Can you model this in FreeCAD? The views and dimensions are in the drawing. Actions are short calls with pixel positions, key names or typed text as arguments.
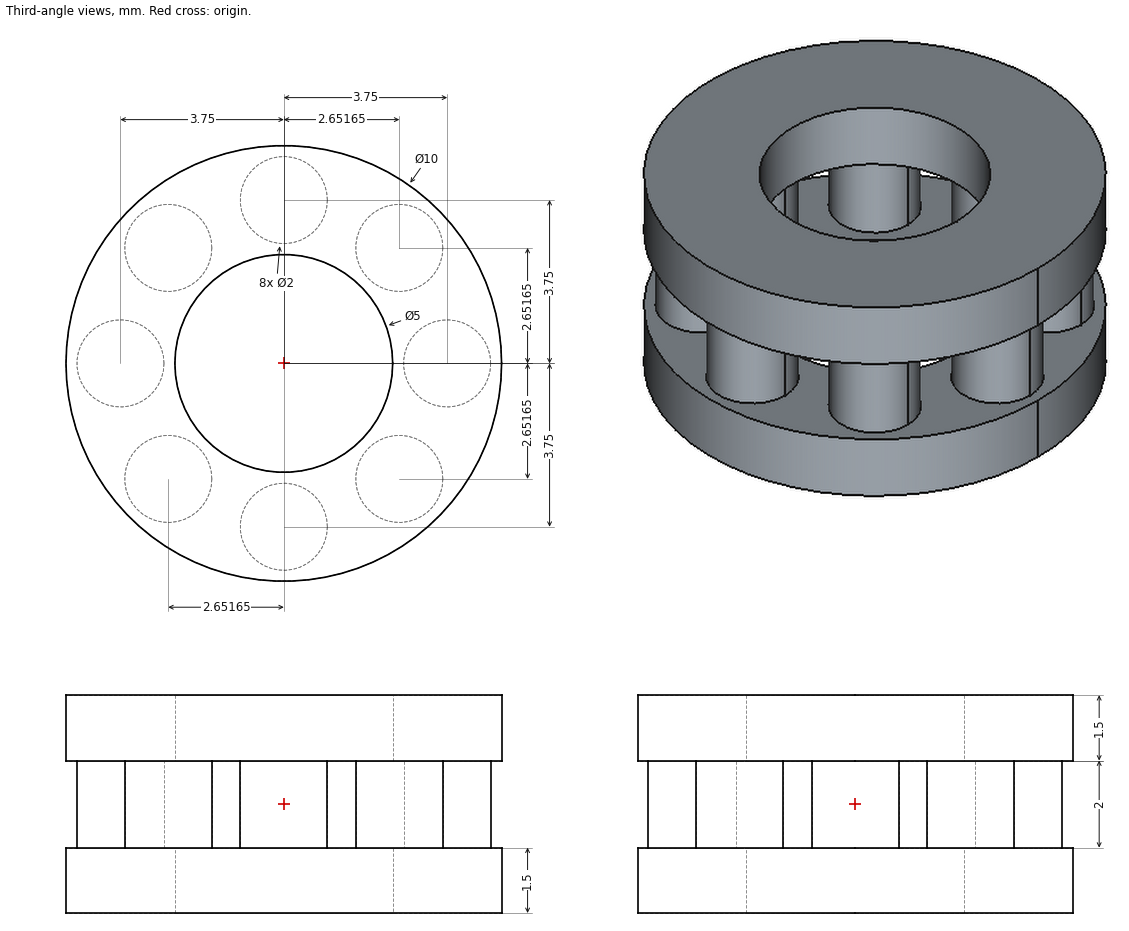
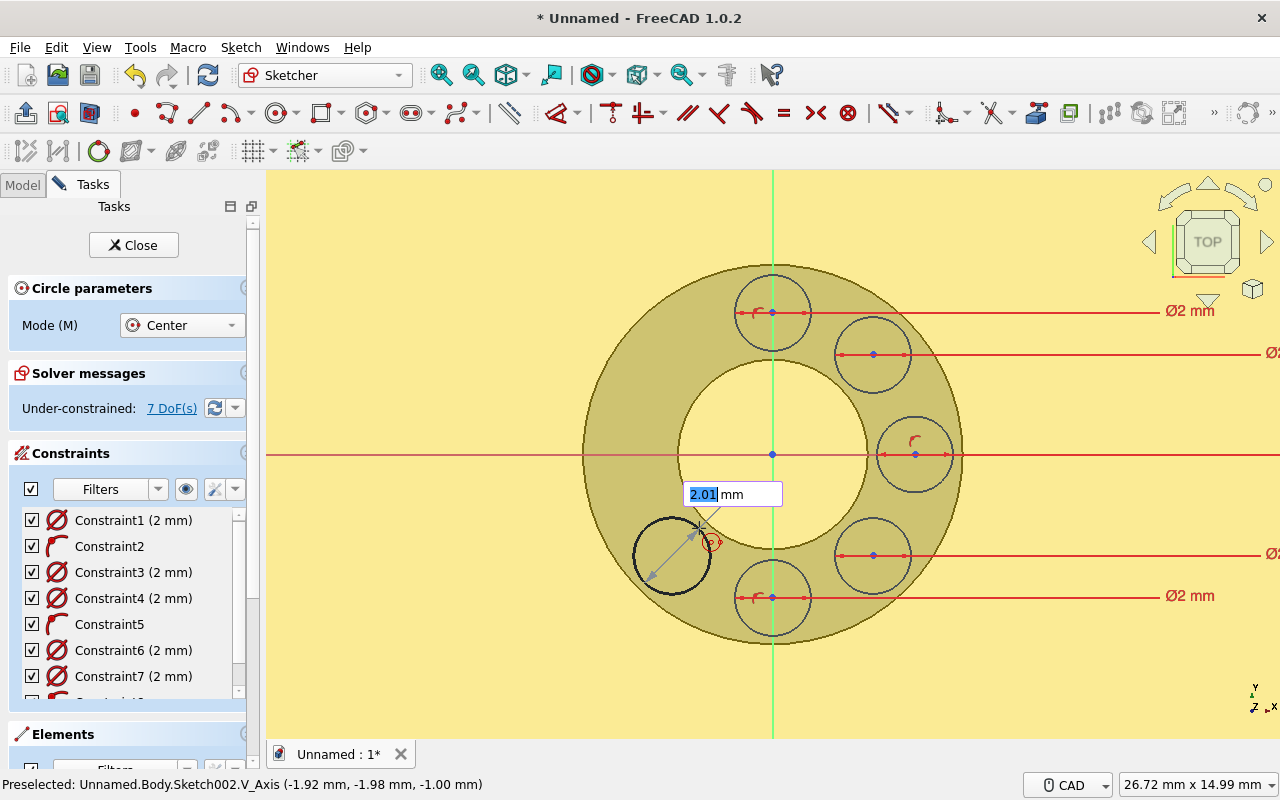
text(2)
key(Return)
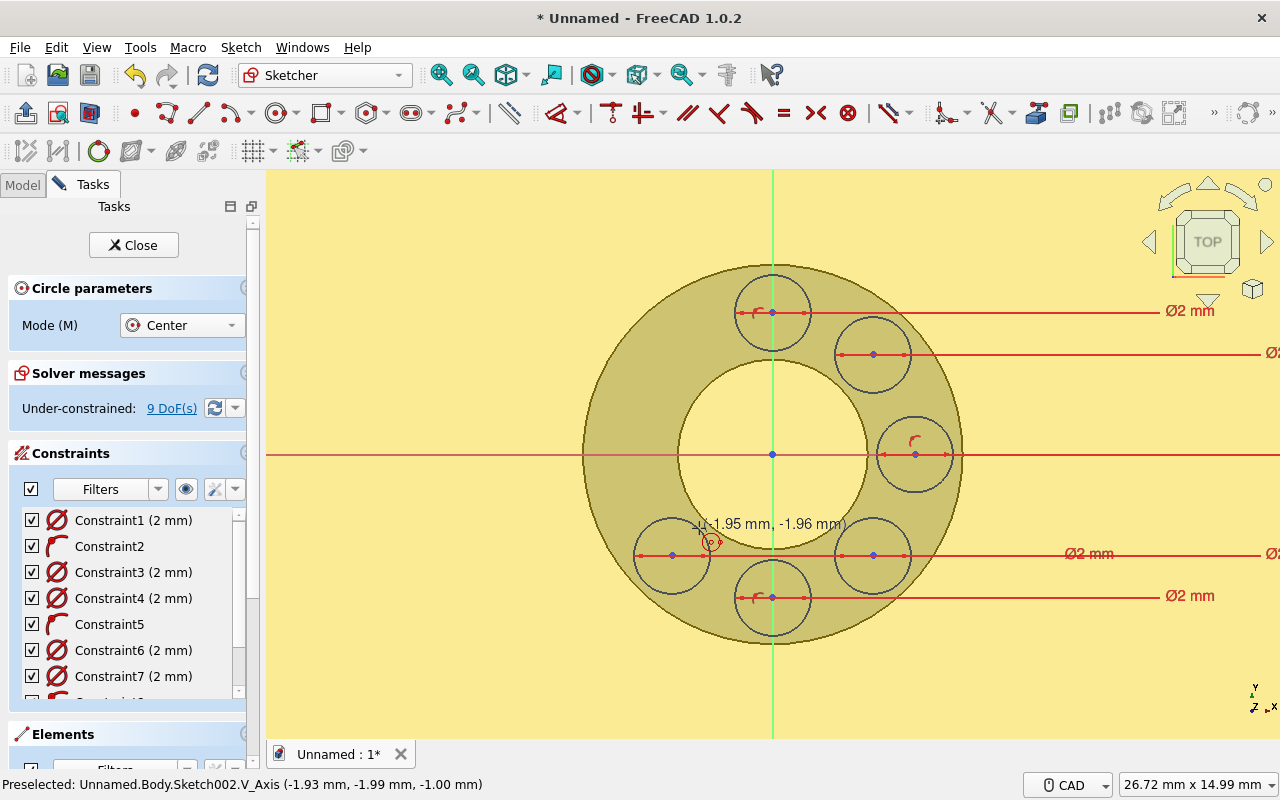
click(631, 454)
move(657, 428)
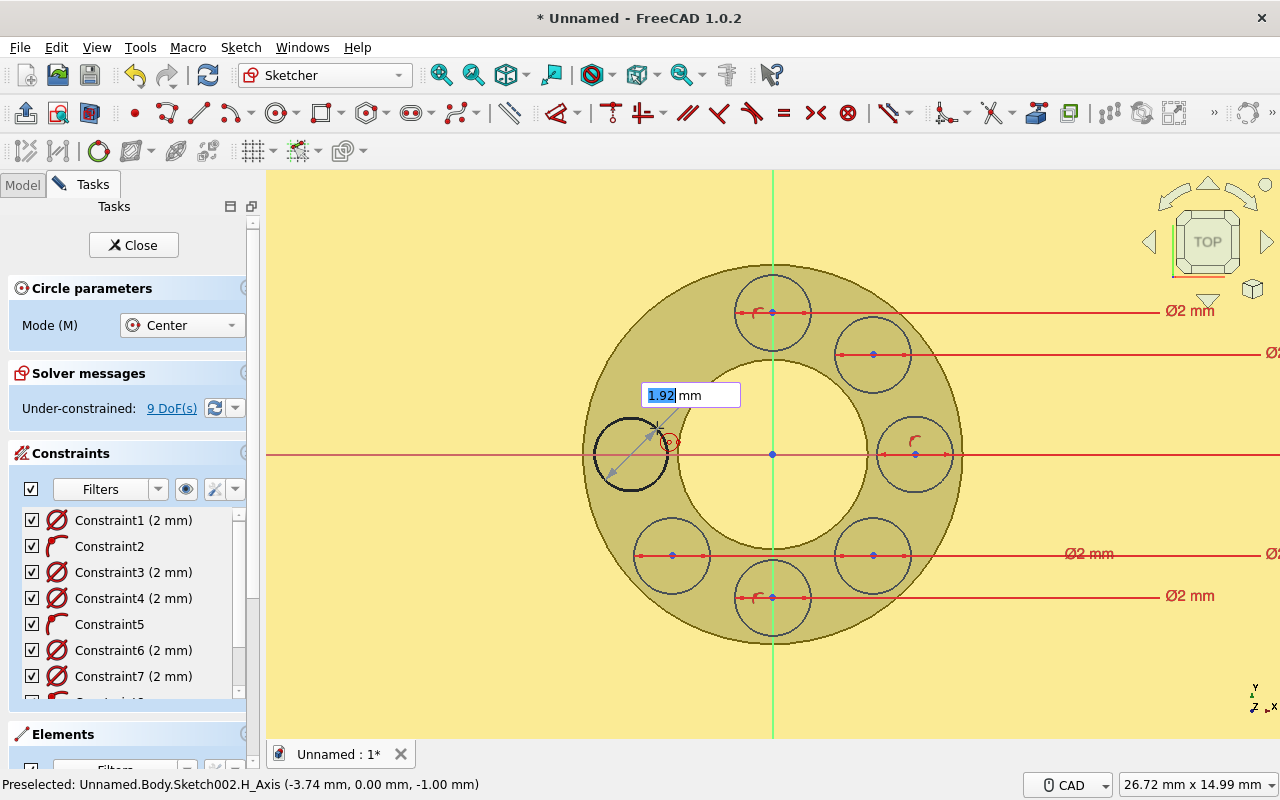
text(2)
key(Return)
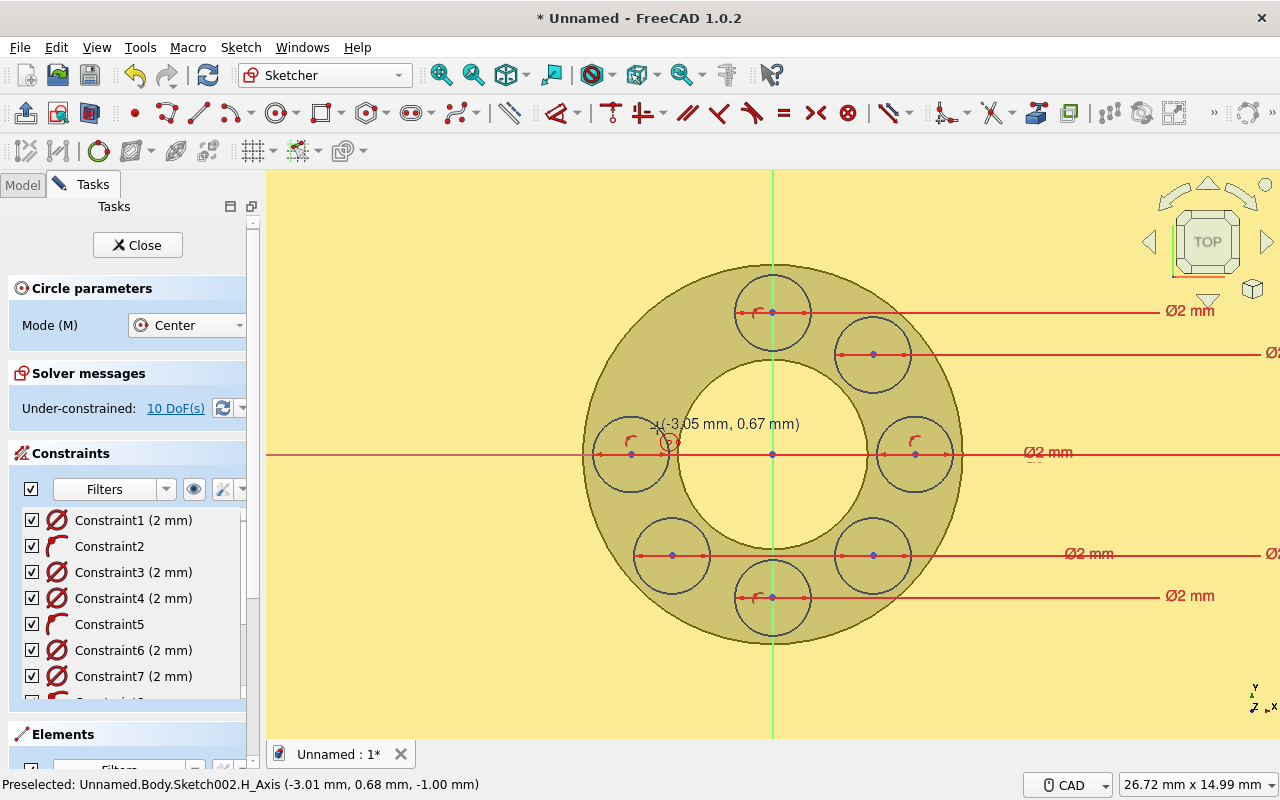
click(672, 354)
move(699, 327)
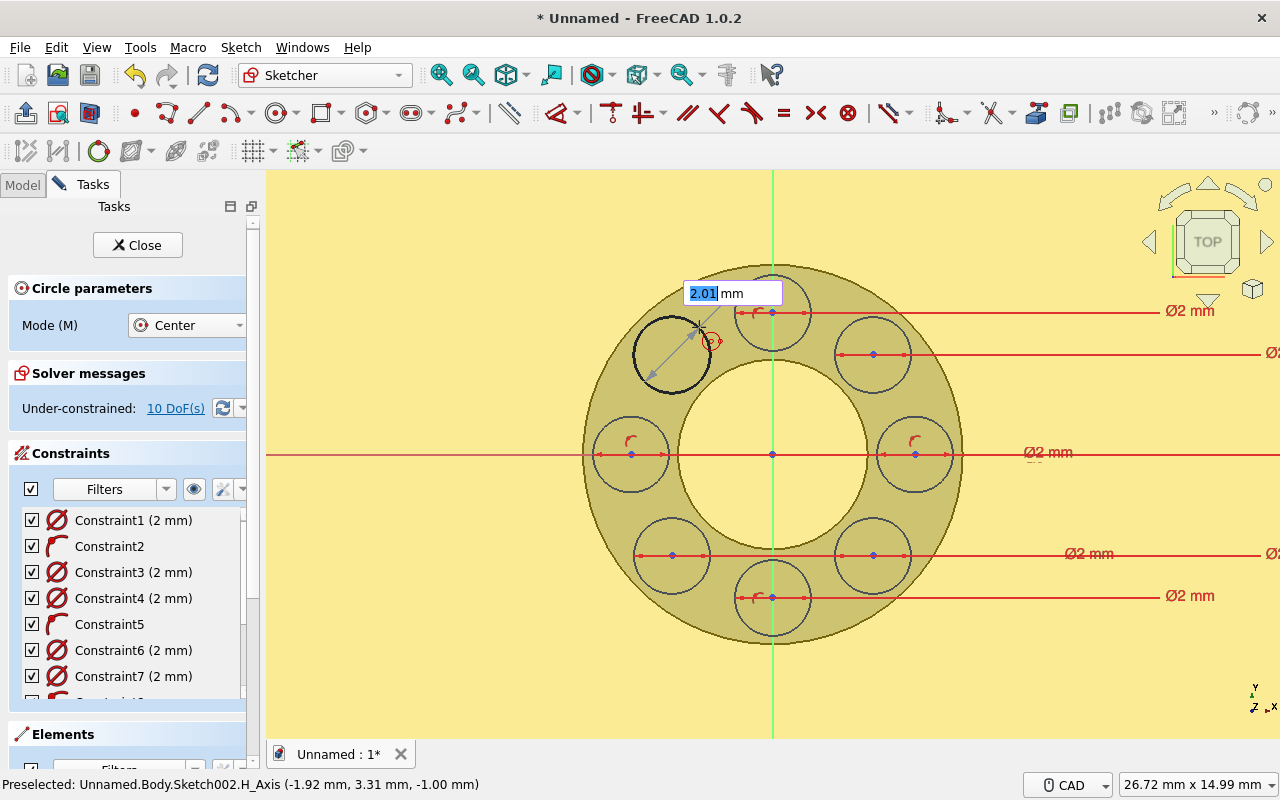
text(2)
key(Return)
key(Escape)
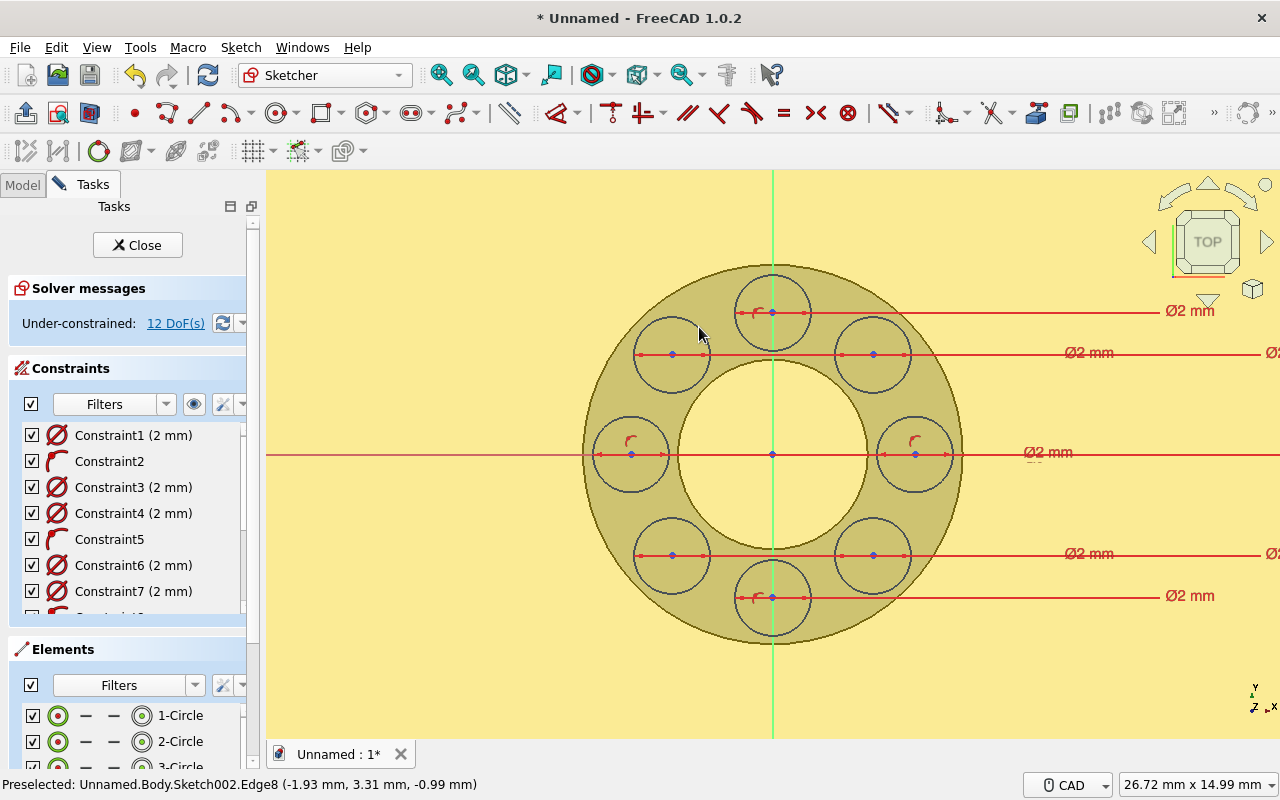
click(873, 355)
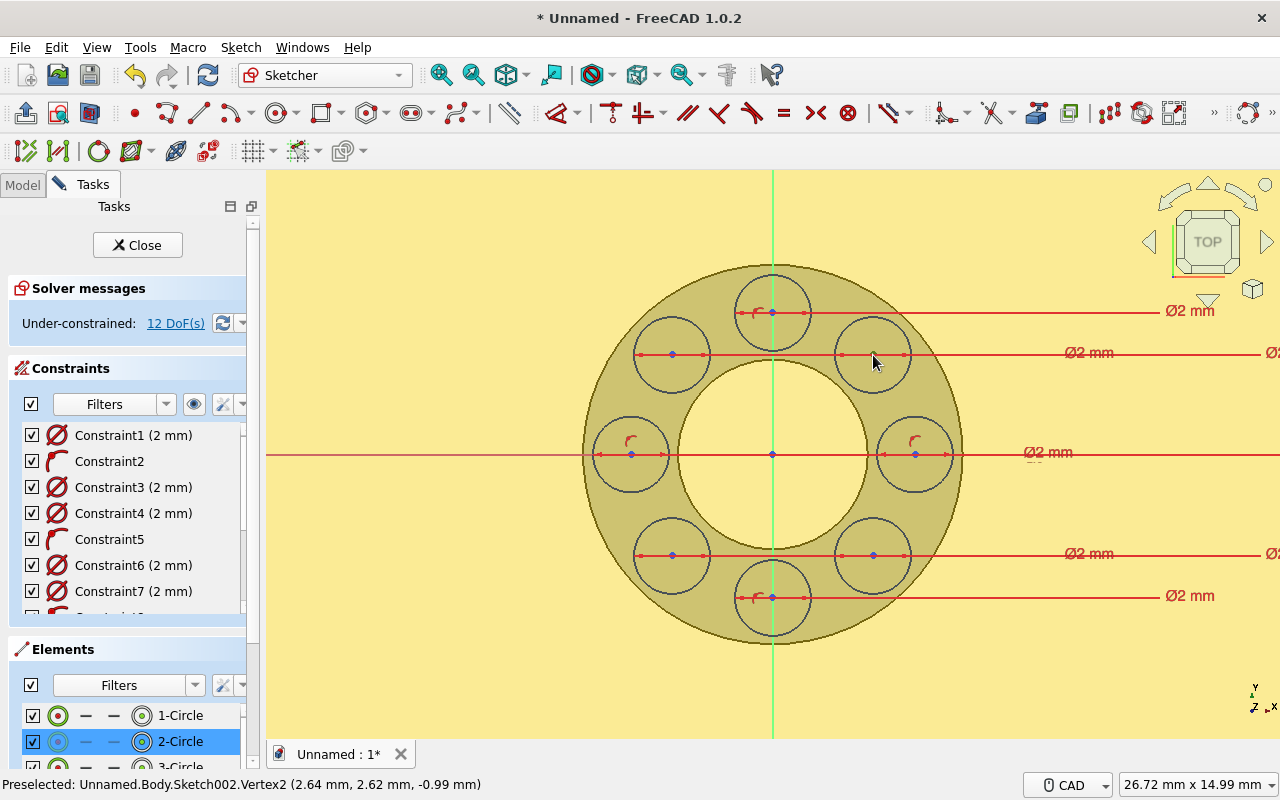
click(873, 556)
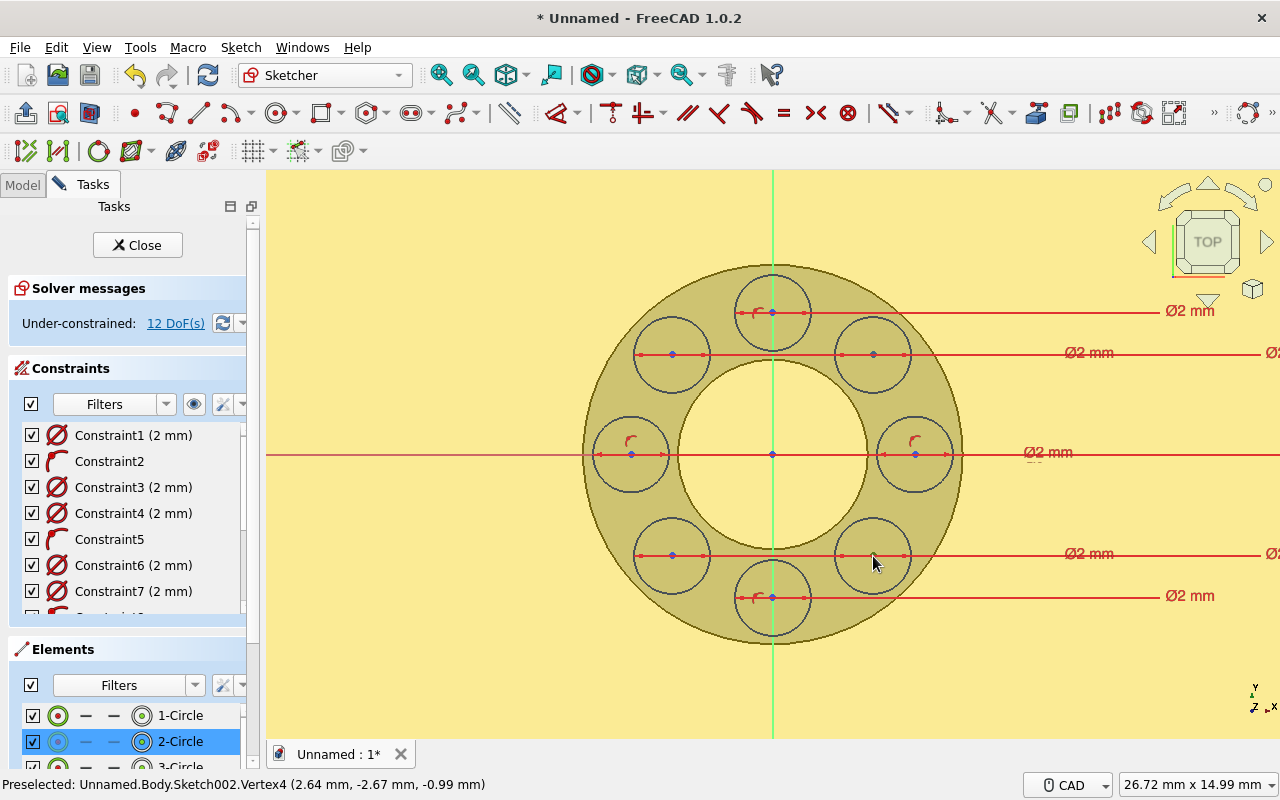
click(666, 114)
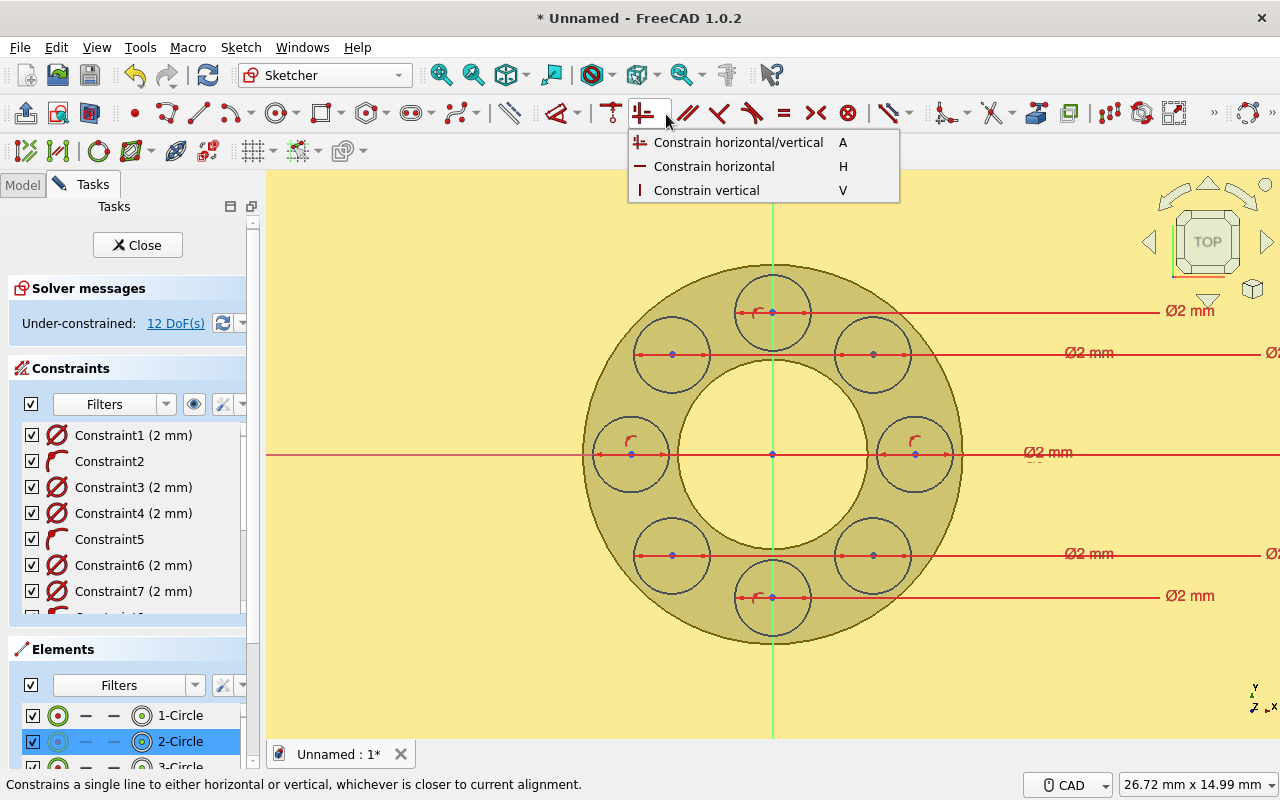
click(764, 190)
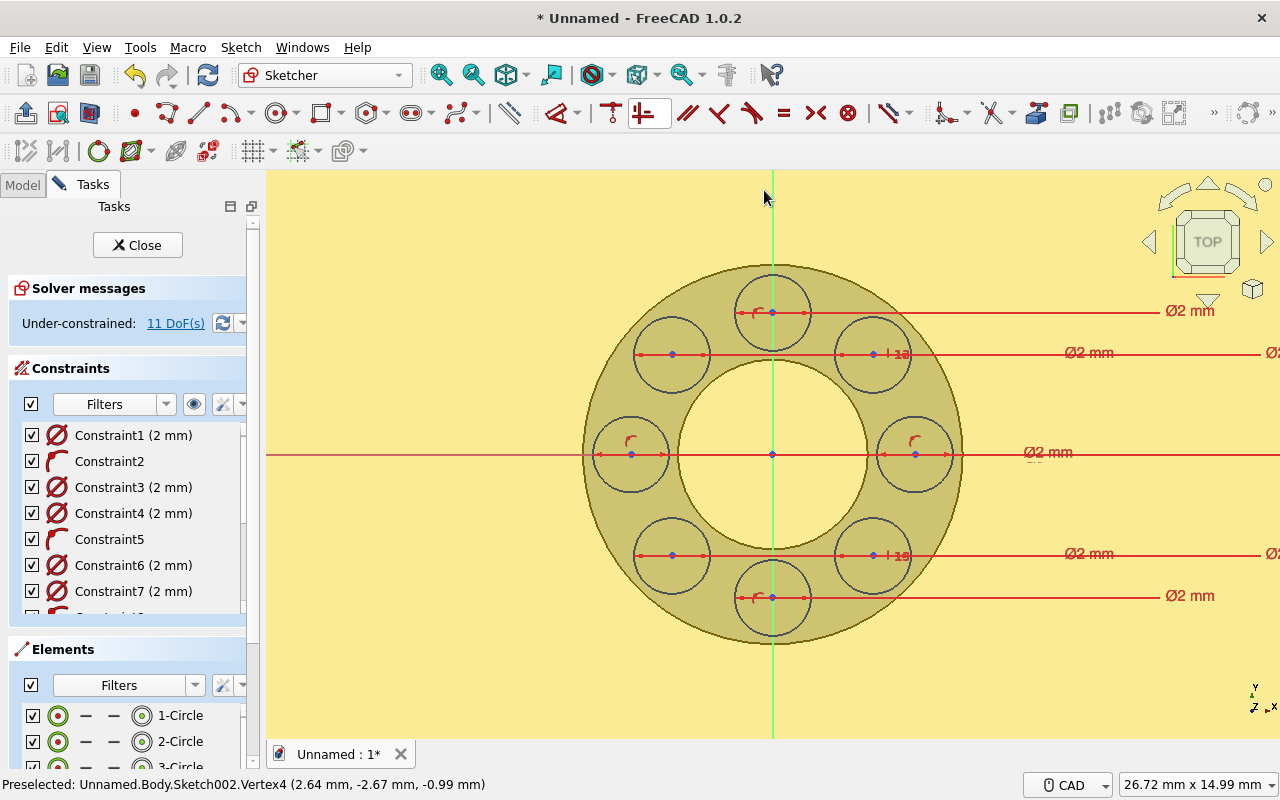
click(873, 556)